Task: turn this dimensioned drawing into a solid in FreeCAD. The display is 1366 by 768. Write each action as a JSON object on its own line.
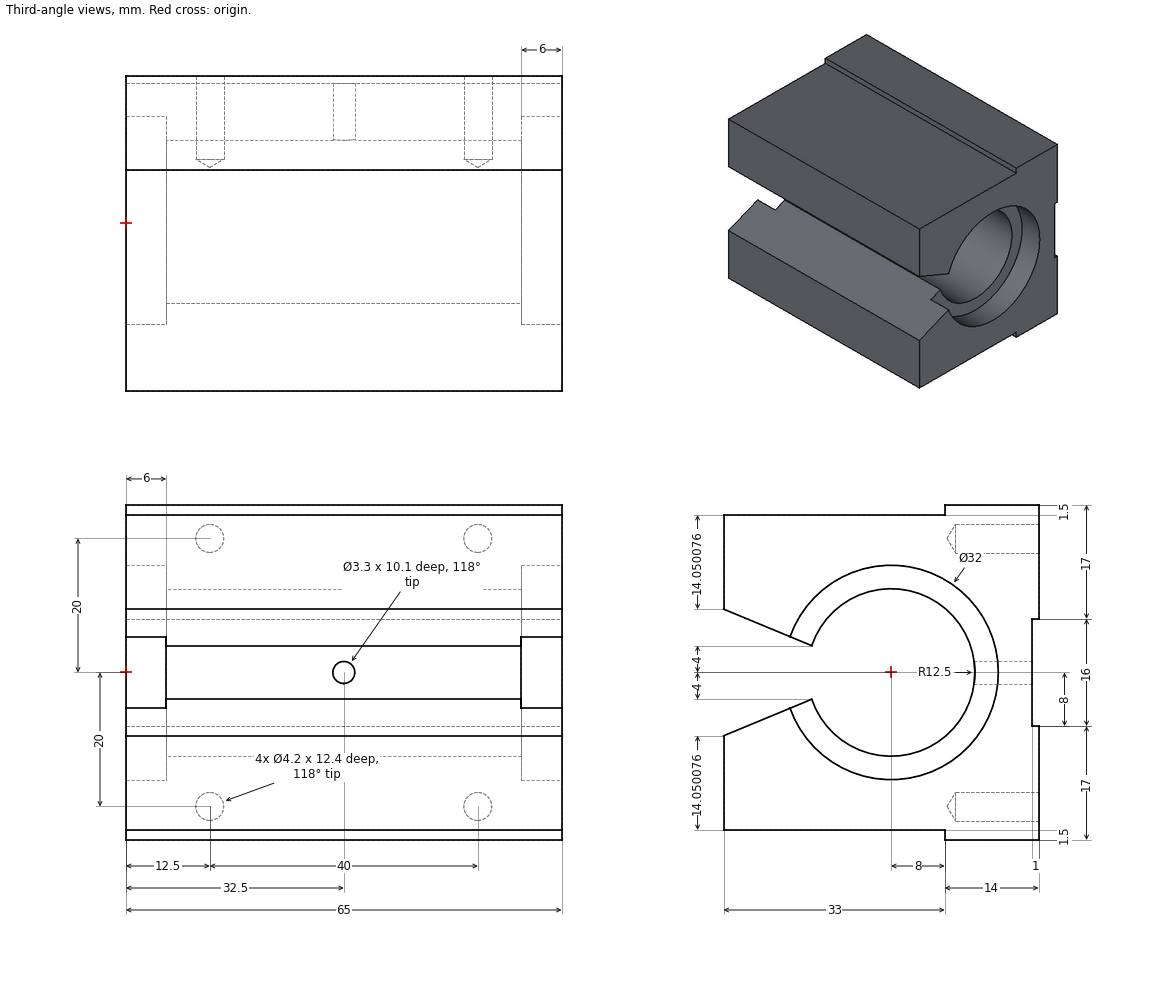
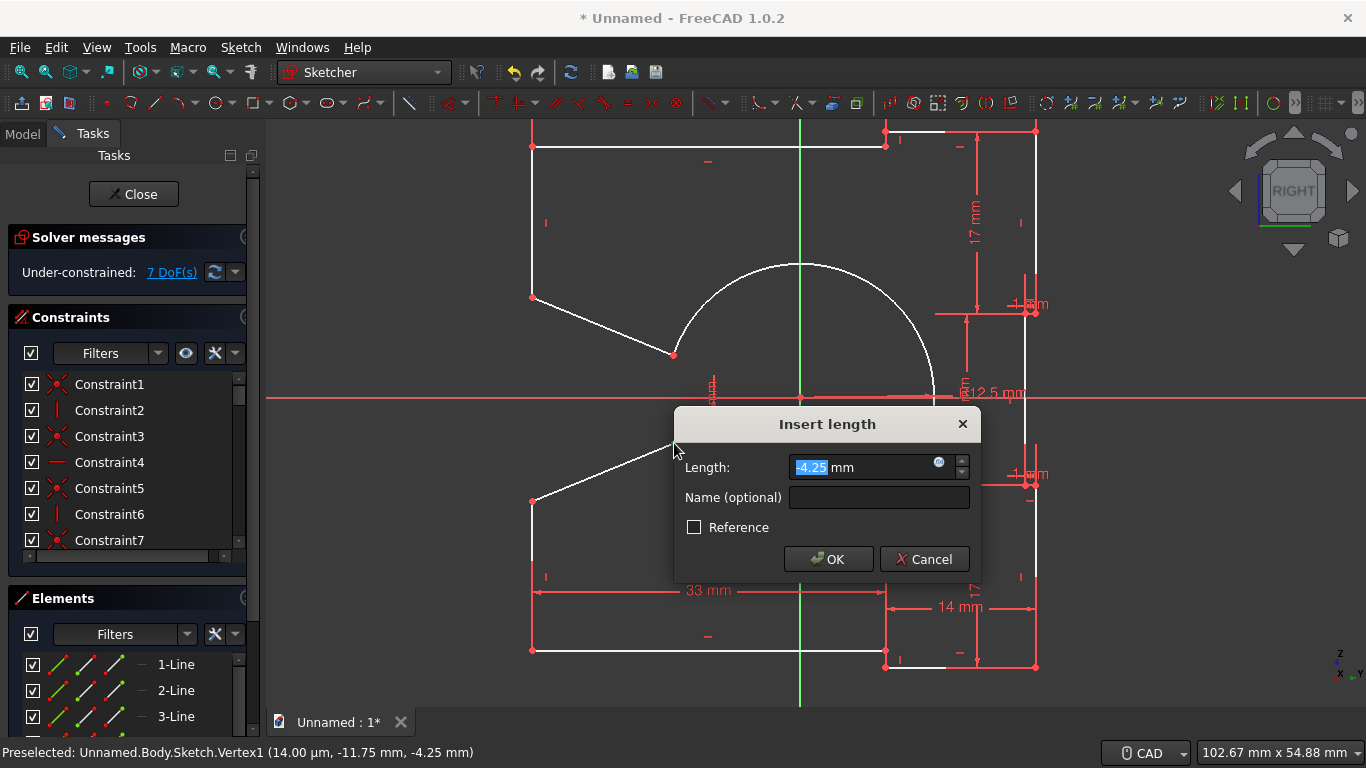
{"action": "type", "text": "-4"}
{"action": "key", "text": "Return"}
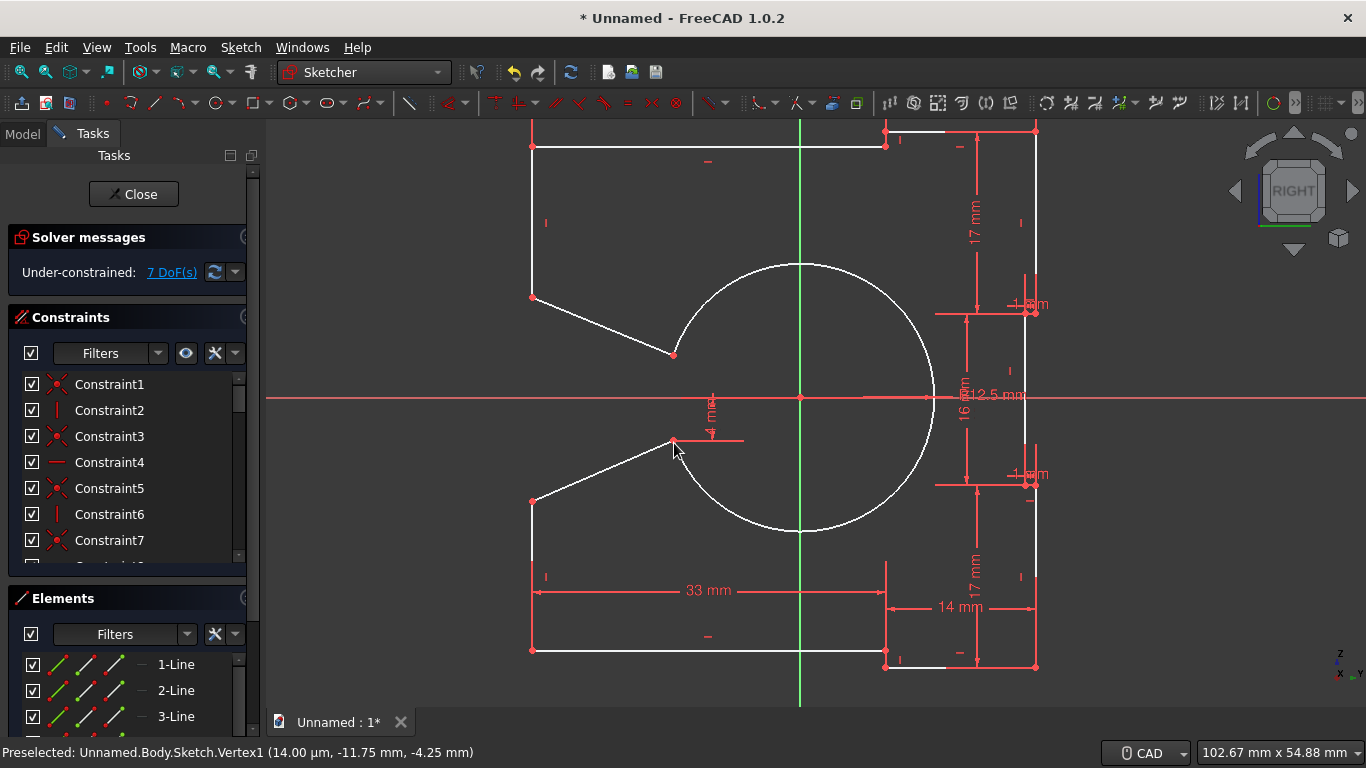
{"action": "left_click", "coordinate": [886, 651]}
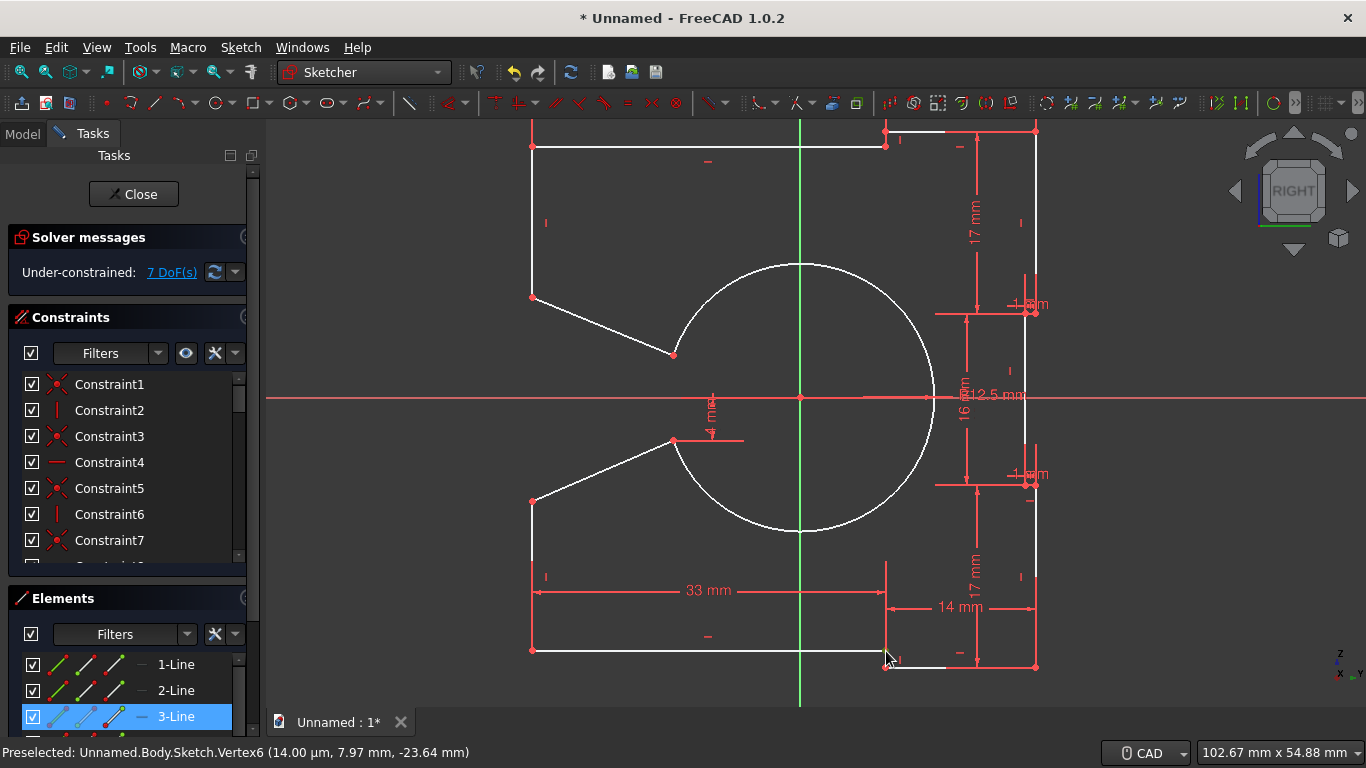
{"action": "left_click", "coordinate": [468, 104]}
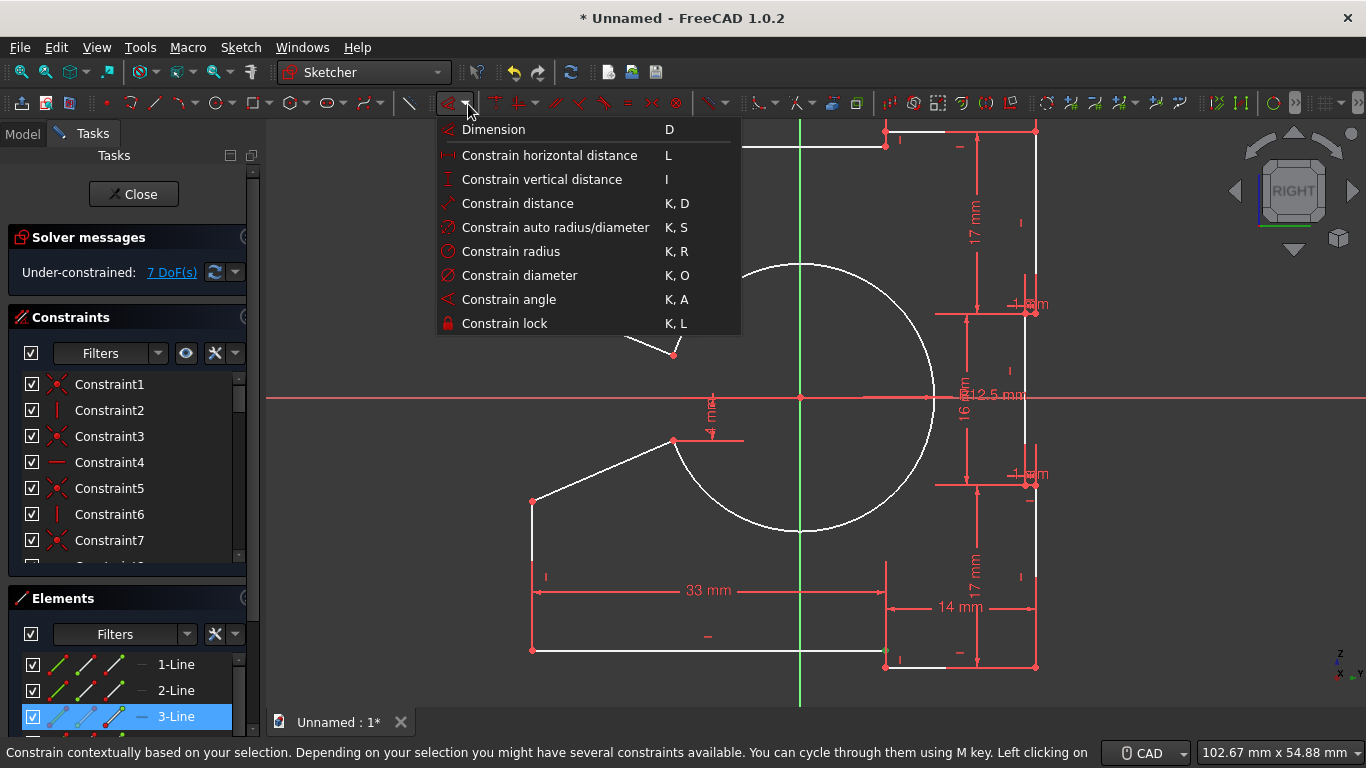
{"action": "left_click", "coordinate": [589, 155]}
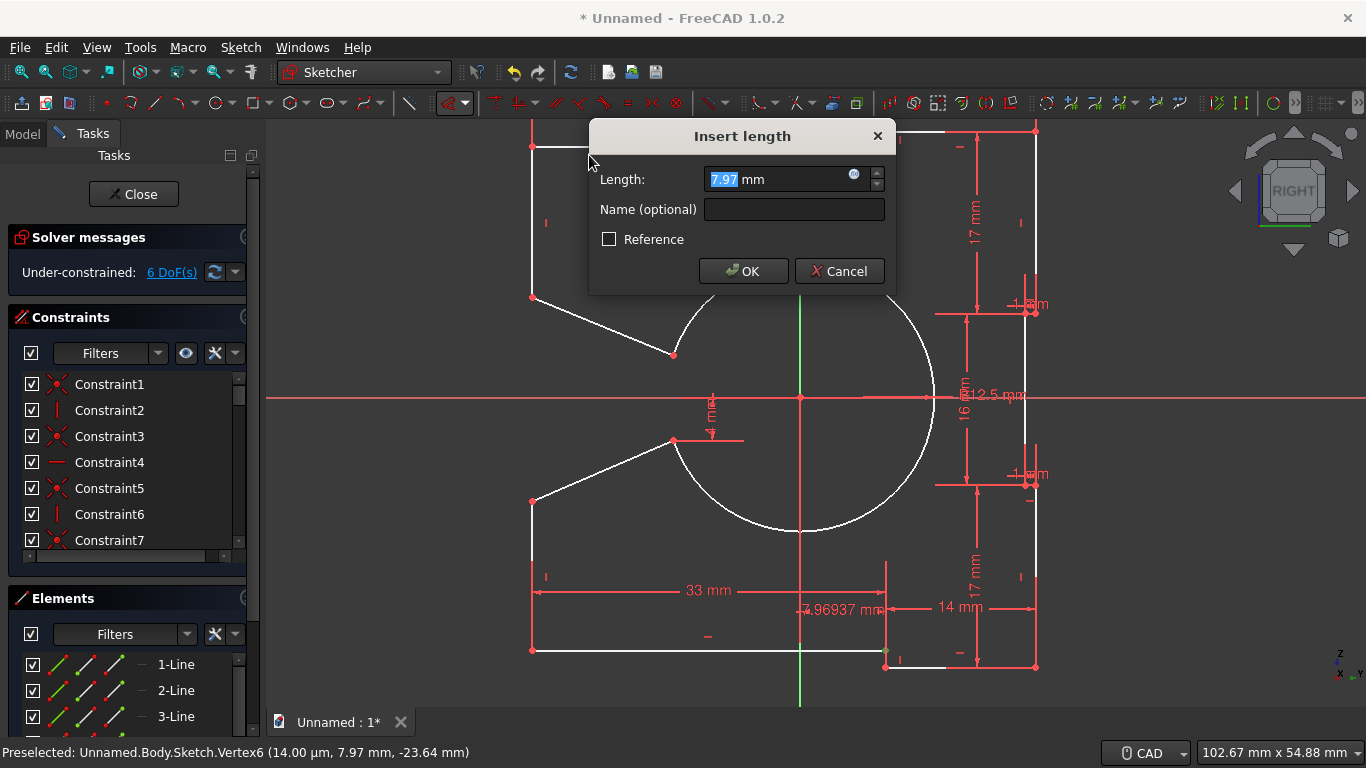
{"action": "type", "text": "8"}
{"action": "key", "text": "Return"}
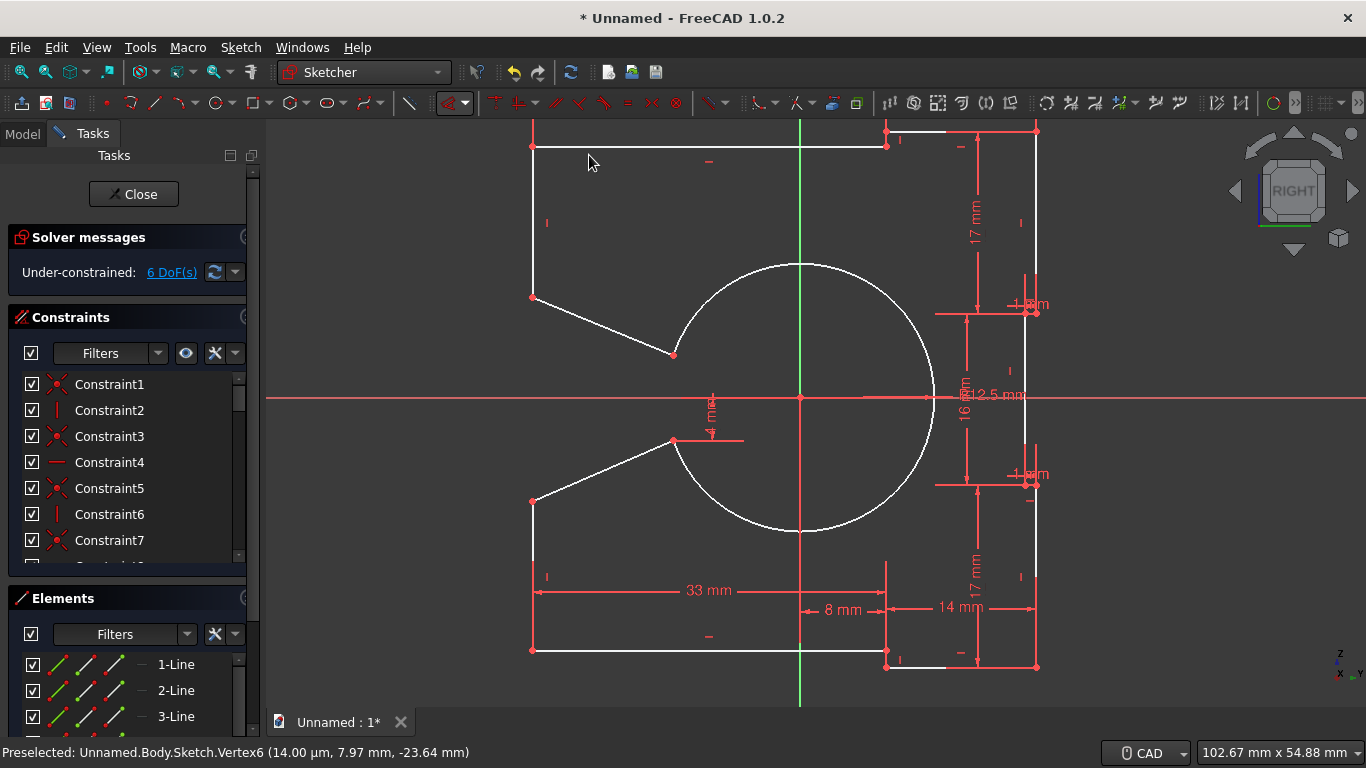
{"action": "left_click", "coordinate": [1036, 485]}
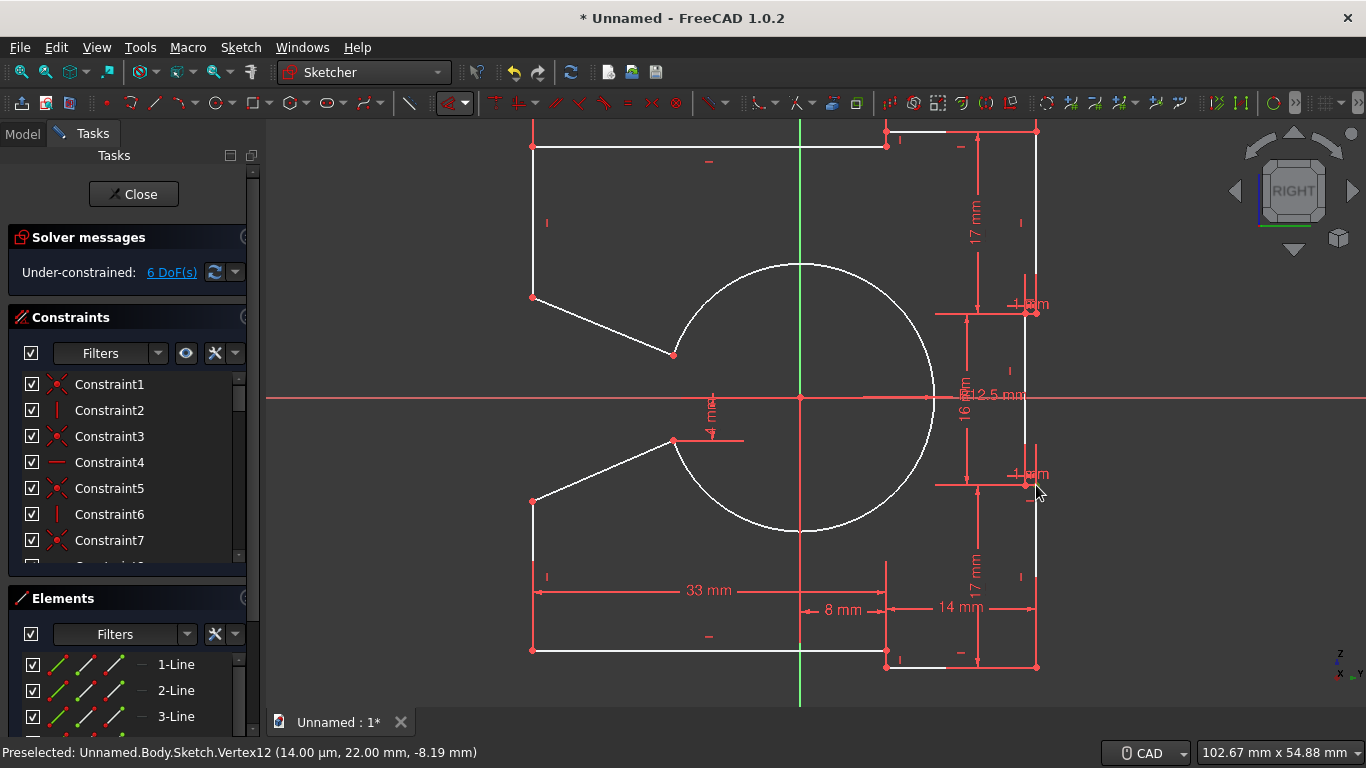
{"action": "key", "text": "i"}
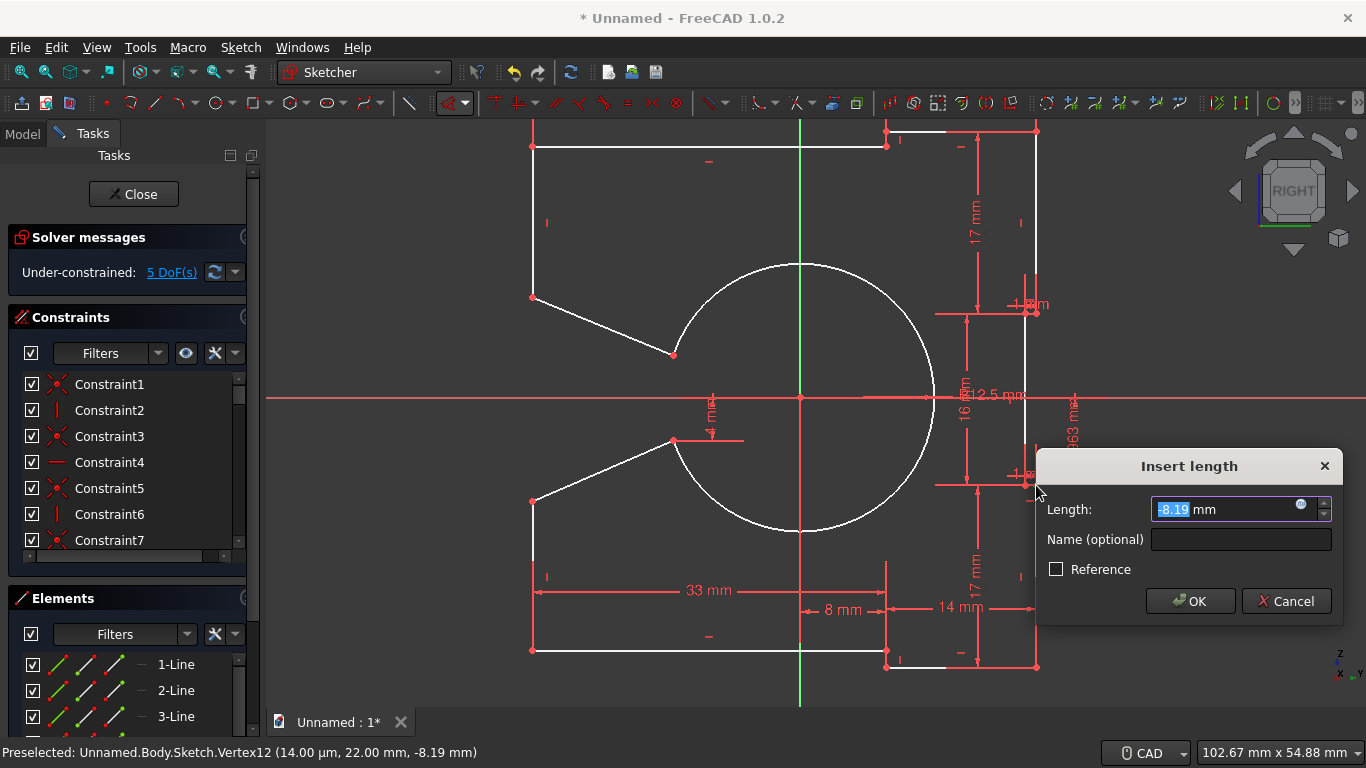
{"action": "type", "text": "-8"}
{"action": "key", "text": "Return"}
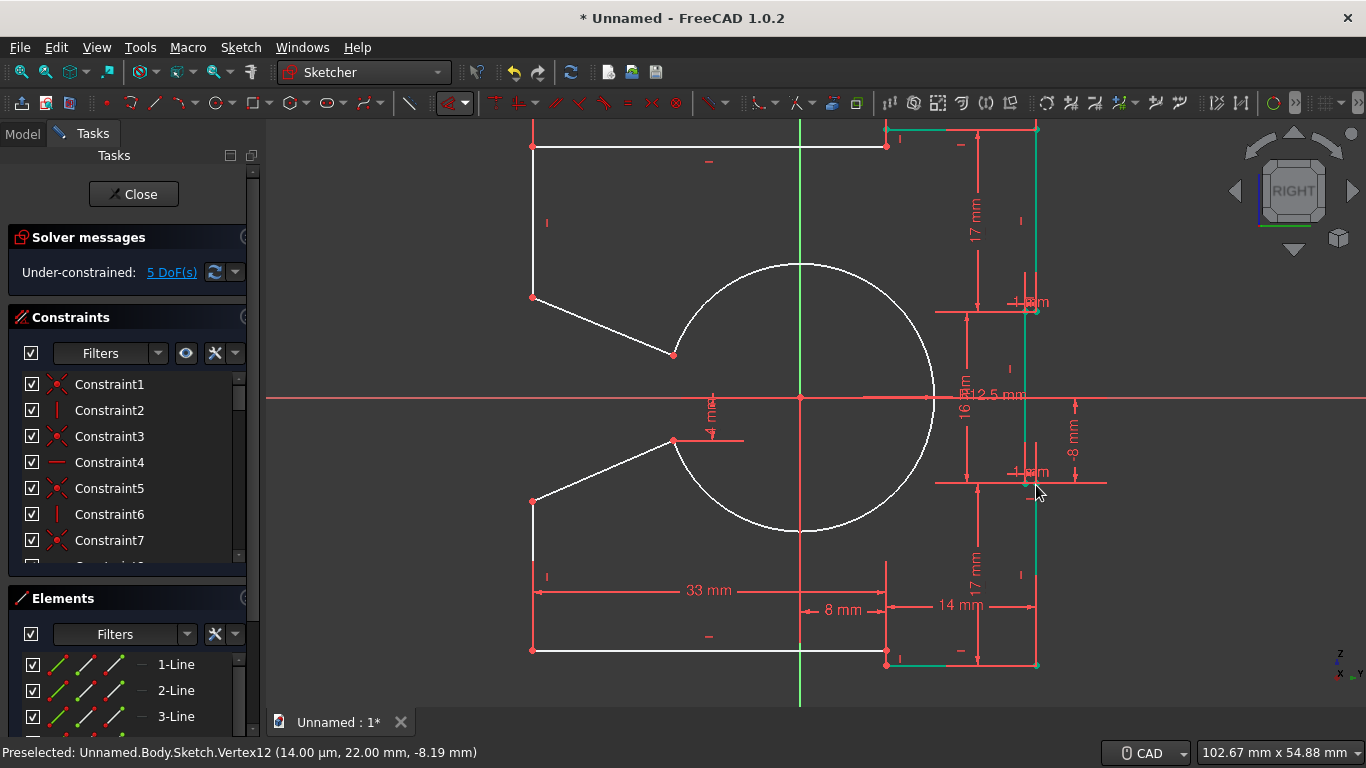
{"action": "left_click", "coordinate": [673, 356]}